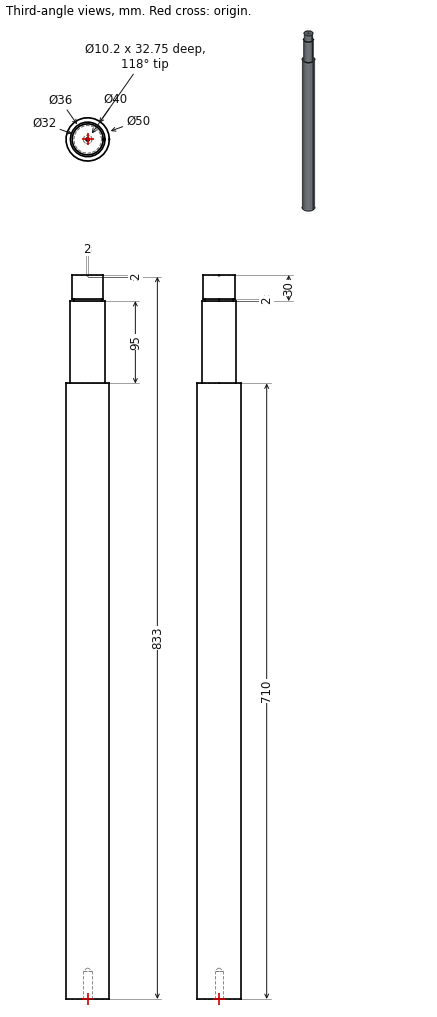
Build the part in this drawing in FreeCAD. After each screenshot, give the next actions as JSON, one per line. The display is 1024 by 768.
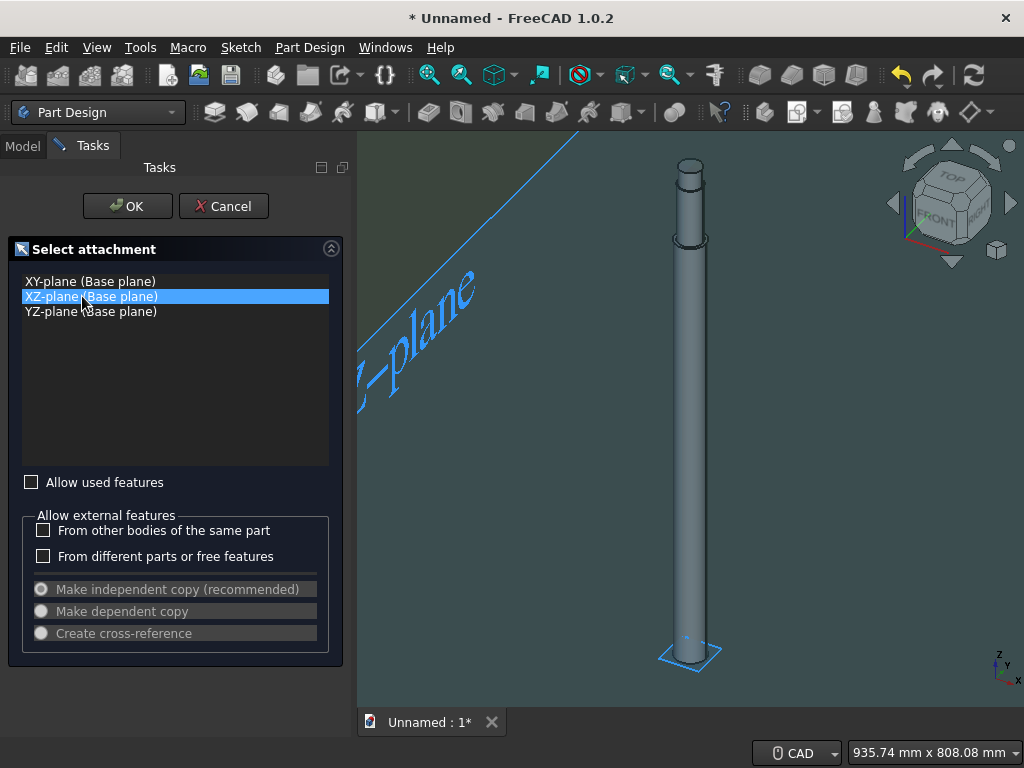
{"action": "left_click", "coordinate": [128, 206]}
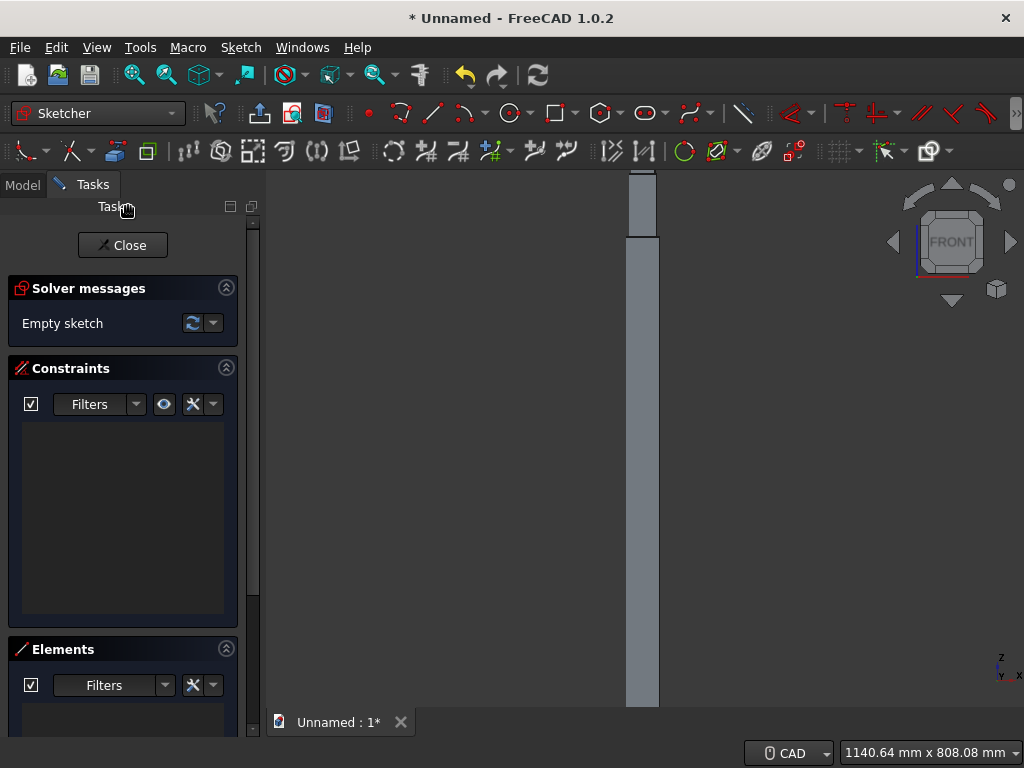
{"action": "left_click", "coordinate": [324, 114]}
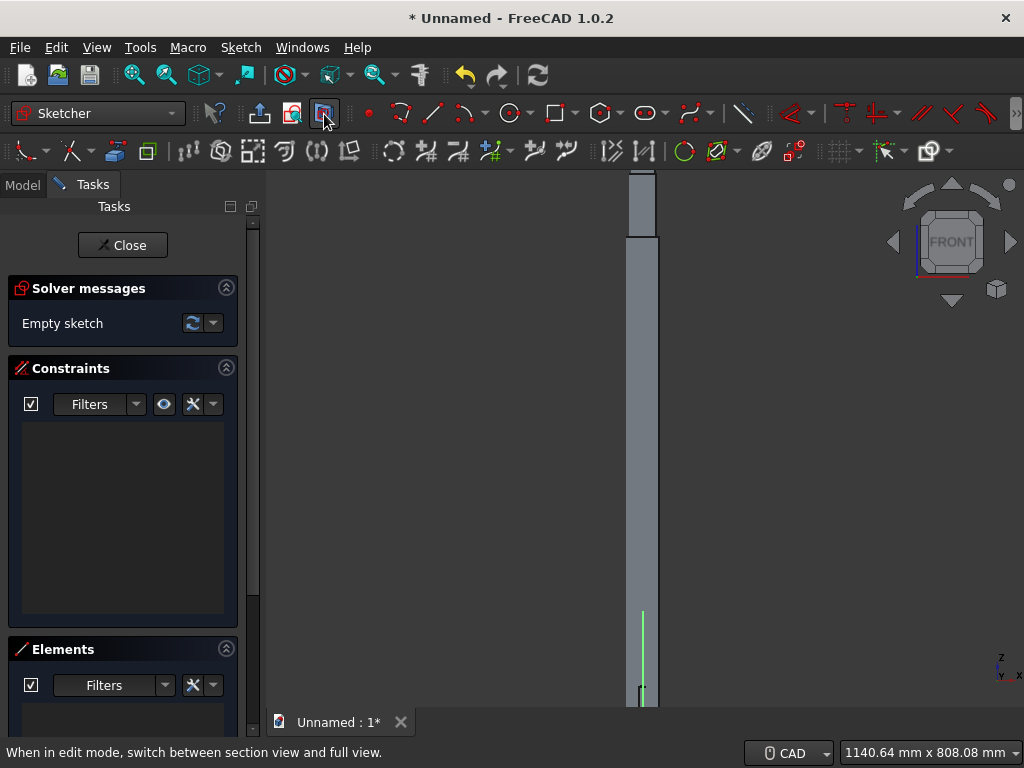
{"action": "scroll", "coordinate": [576, 438], "scroll_direction": "down", "scroll_amount": 5}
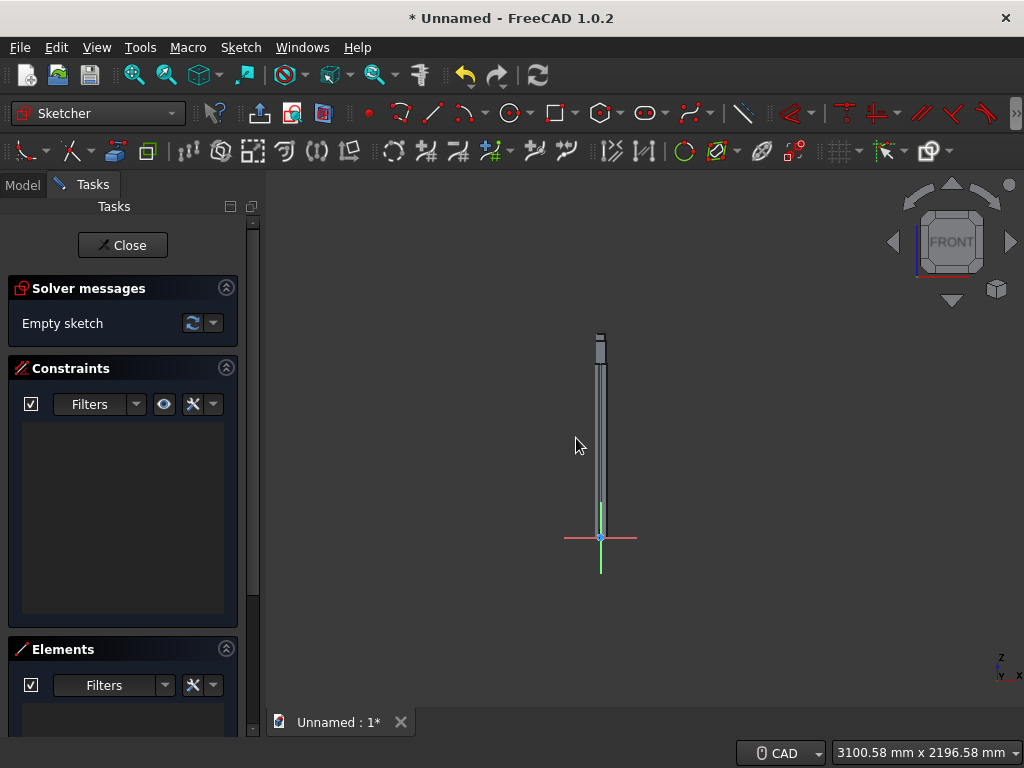
{"action": "scroll", "coordinate": [602, 329], "scroll_direction": "up", "scroll_amount": 15}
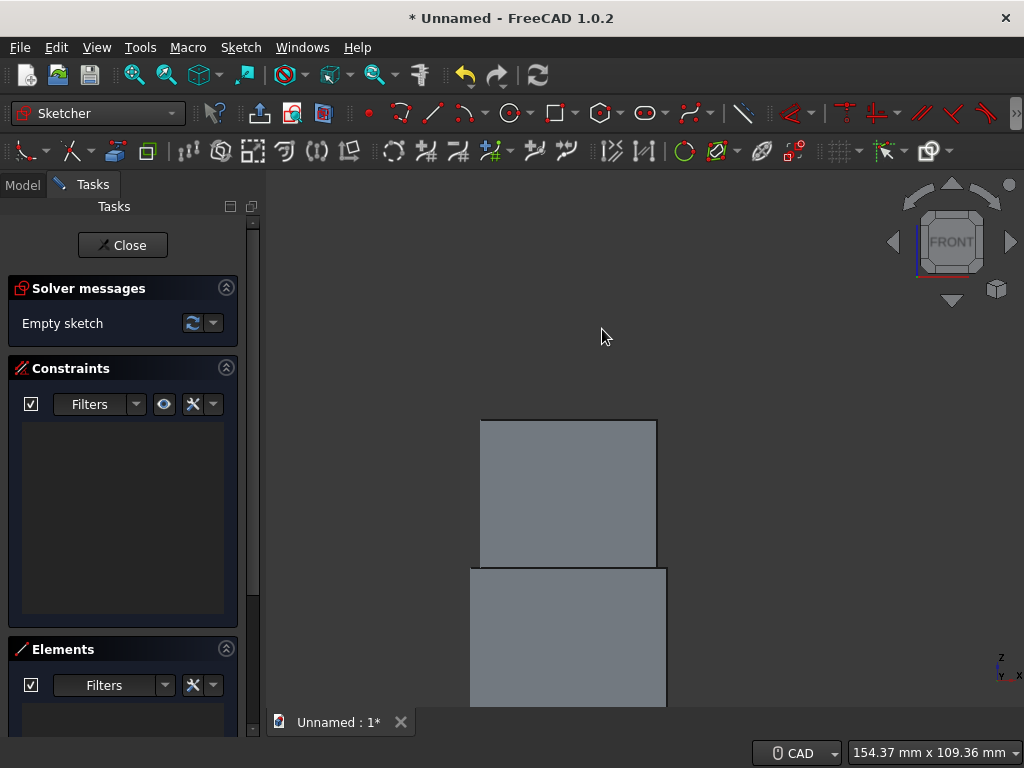
{"action": "scroll", "coordinate": [563, 425], "scroll_direction": "up", "scroll_amount": 15}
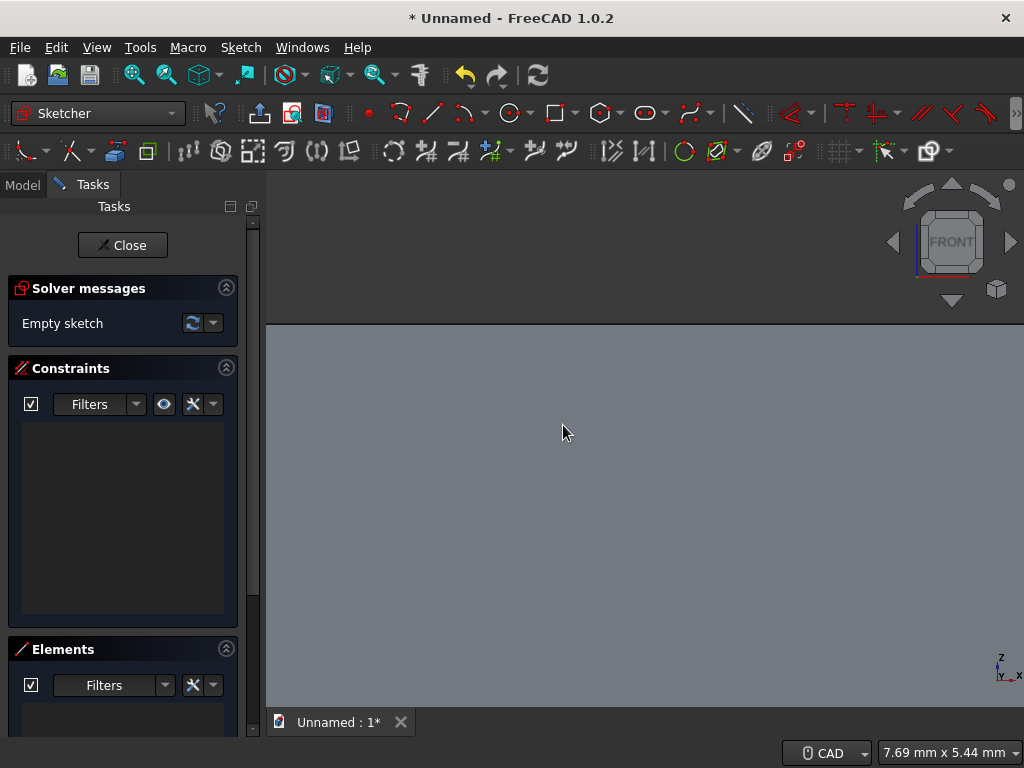
{"action": "scroll", "coordinate": [563, 404], "scroll_direction": "up", "scroll_amount": 3}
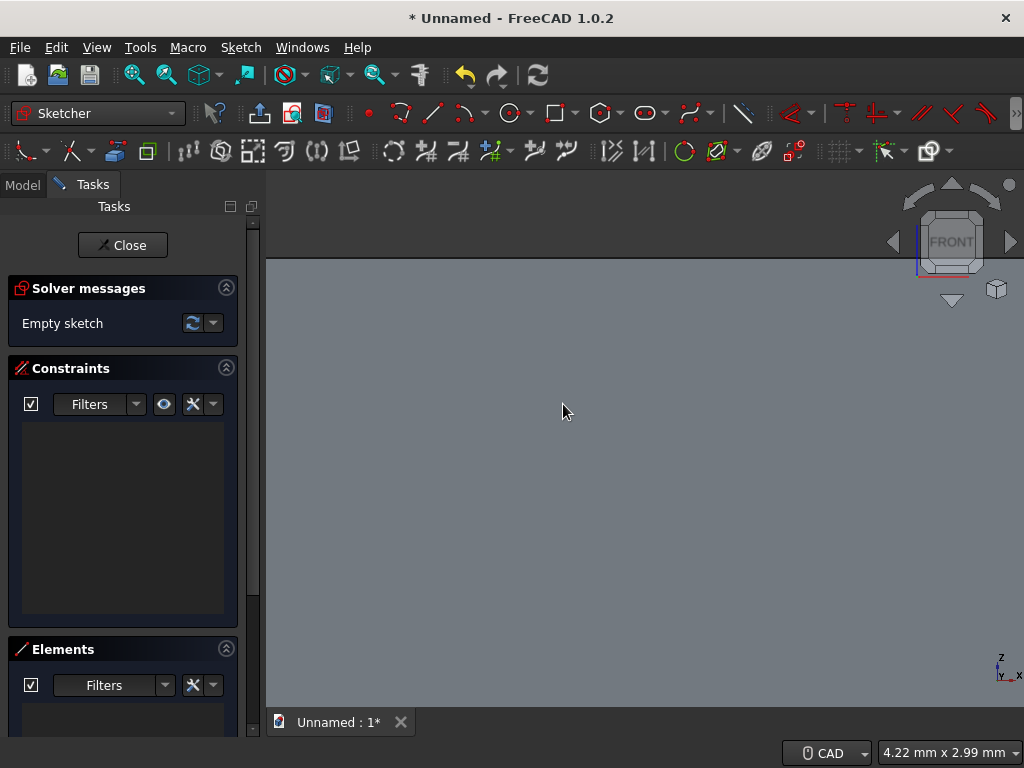
{"action": "left_click", "coordinate": [402, 114]}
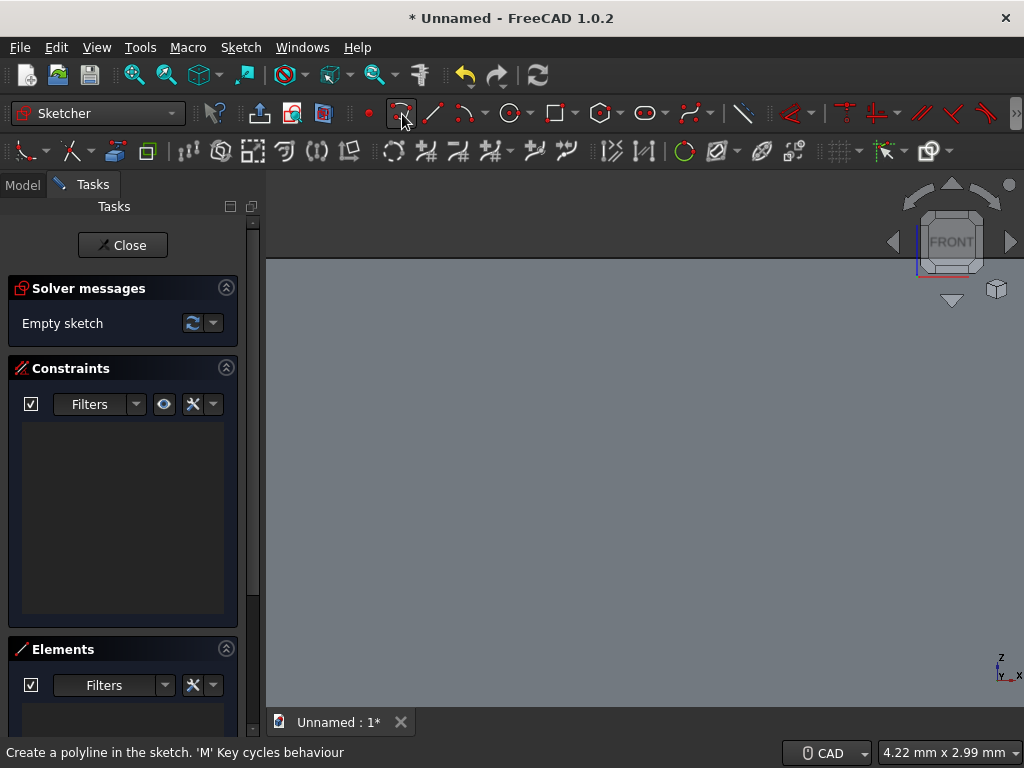
{"action": "left_click", "coordinate": [756, 617]}
{"action": "left_click", "coordinate": [397, 258]}
{"action": "left_click", "coordinate": [747, 258]}
{"action": "left_click", "coordinate": [756, 618]}
{"action": "key", "text": "Escape"}
{"action": "key", "text": "Escape"}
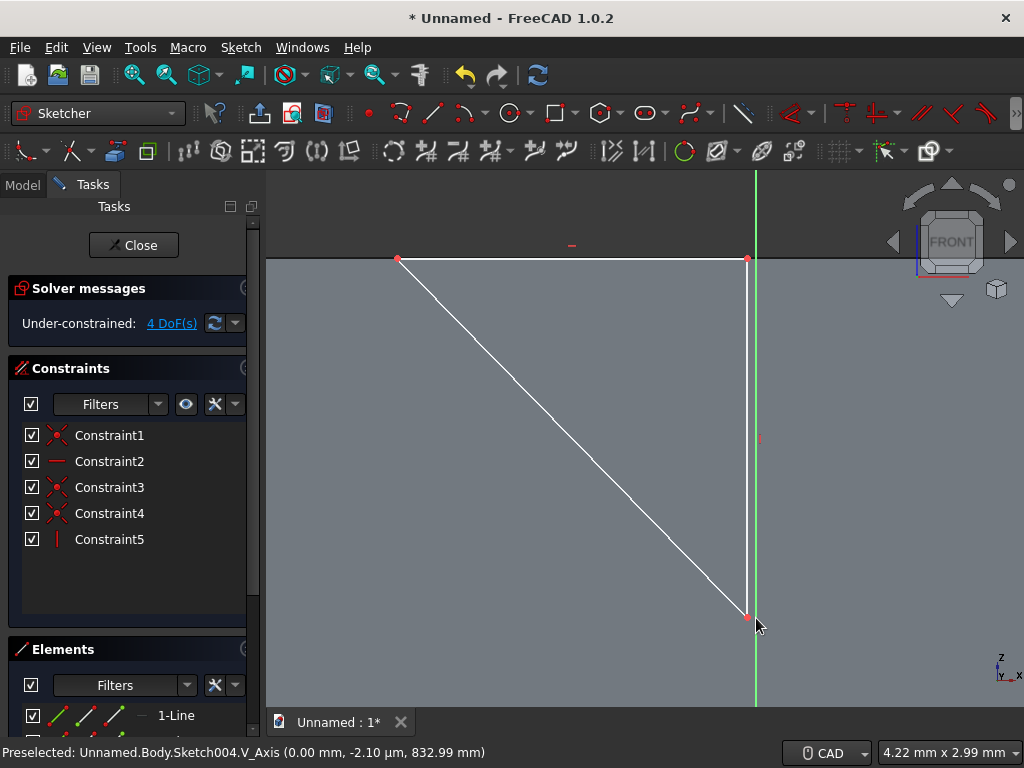
{"action": "left_click", "coordinate": [747, 618]}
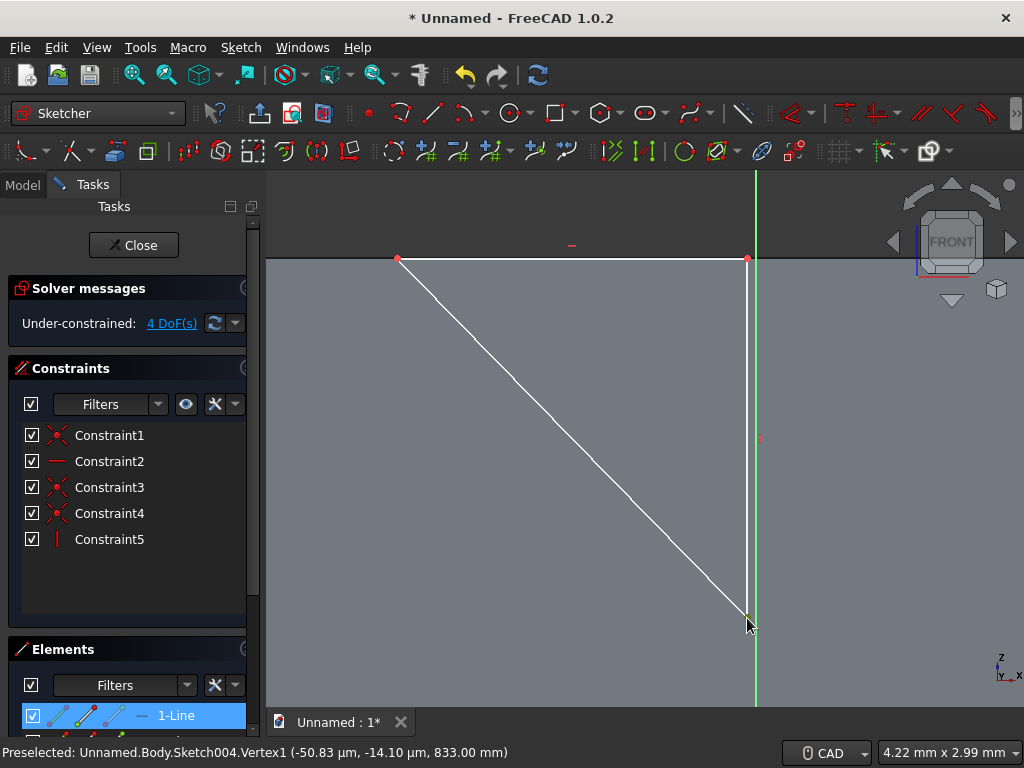
{"action": "left_click", "coordinate": [756, 232]}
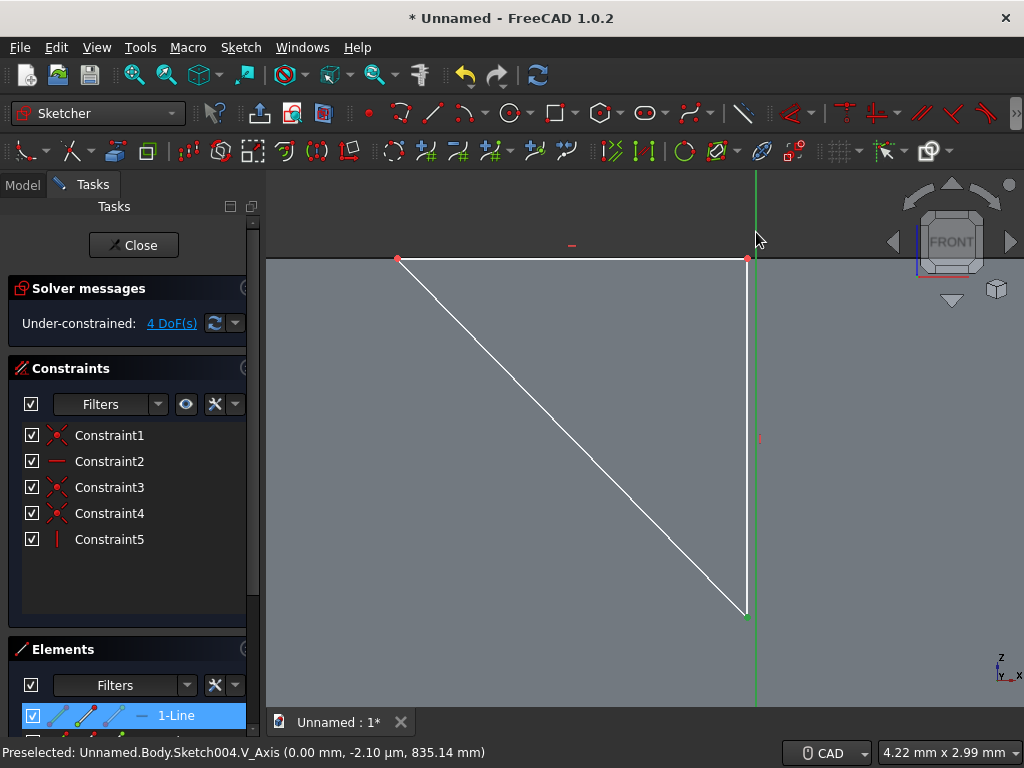
{"action": "left_click", "coordinate": [846, 114]}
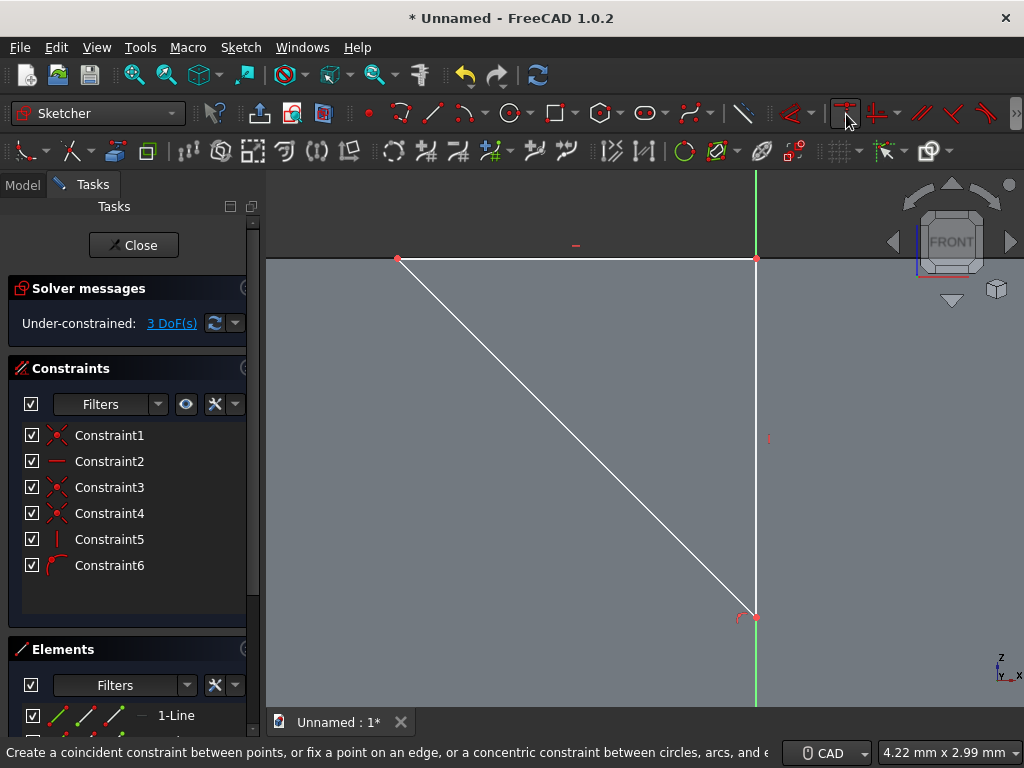
{"action": "left_click", "coordinate": [790, 114]}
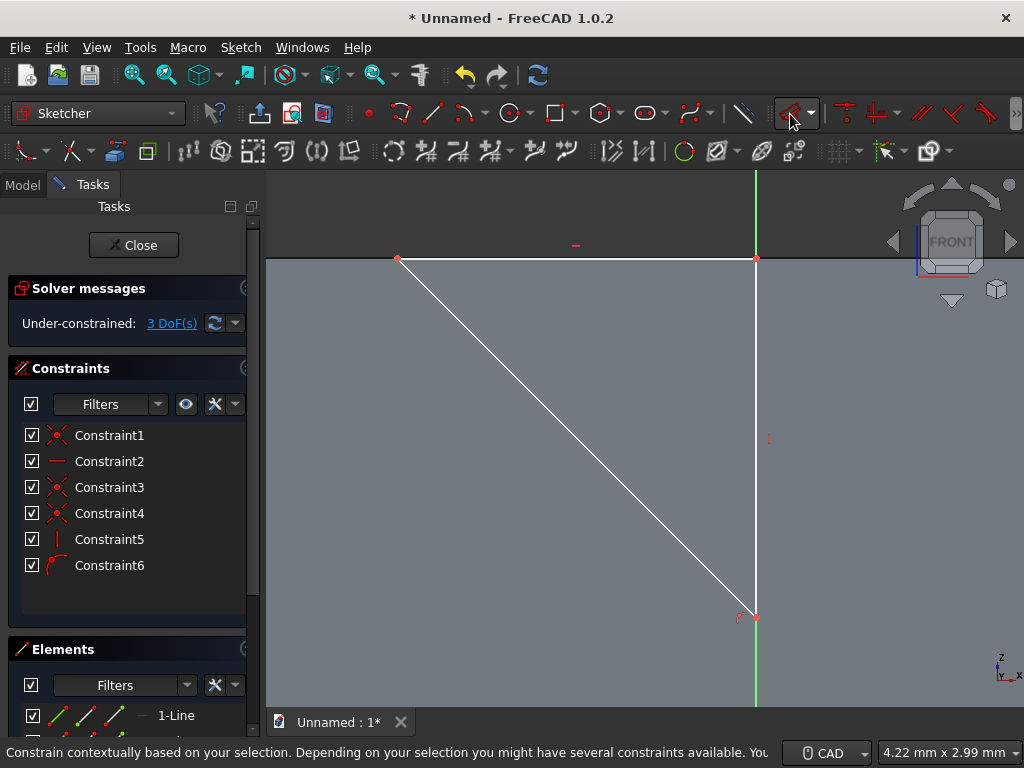
{"action": "left_click", "coordinate": [505, 259]}
{"action": "left_click", "coordinate": [577, 225]}